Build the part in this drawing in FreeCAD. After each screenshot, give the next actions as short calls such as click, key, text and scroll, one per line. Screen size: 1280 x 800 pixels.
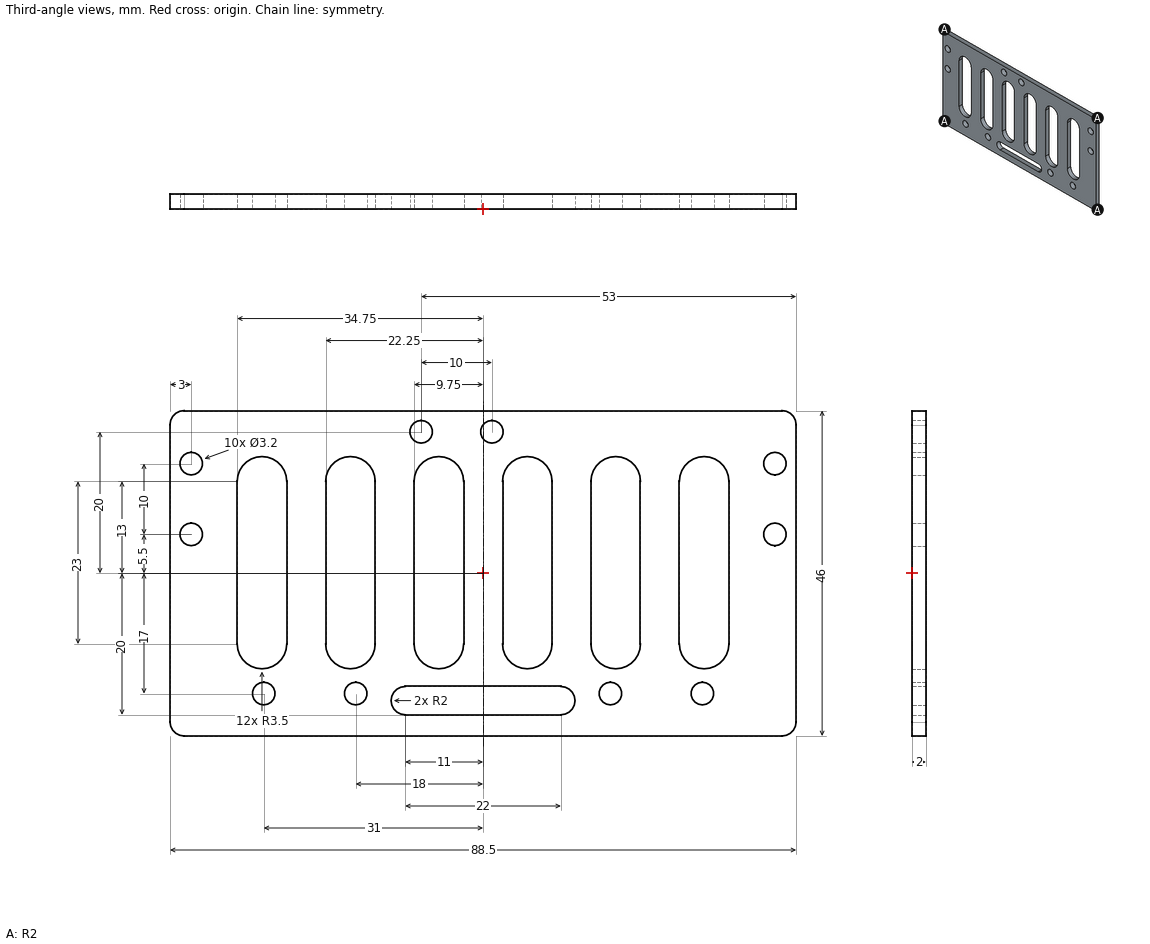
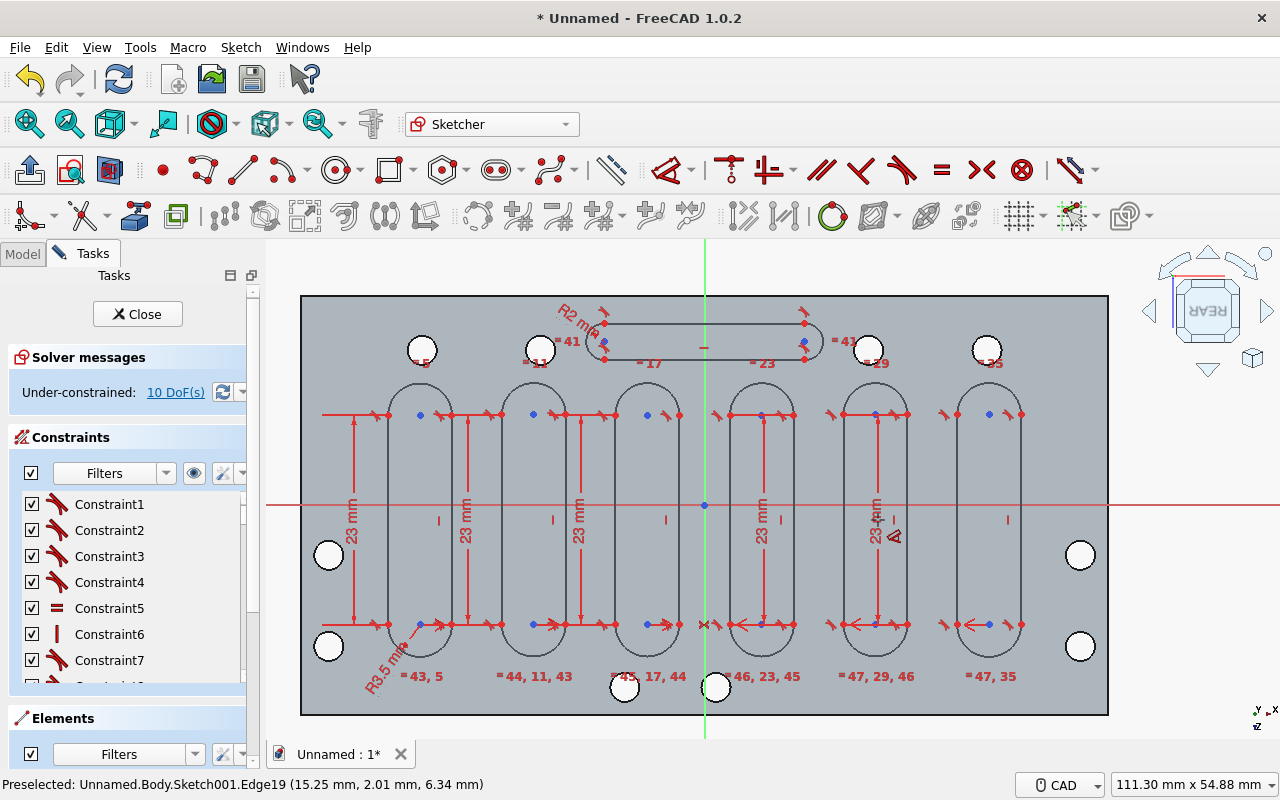
click(957, 562)
click(991, 520)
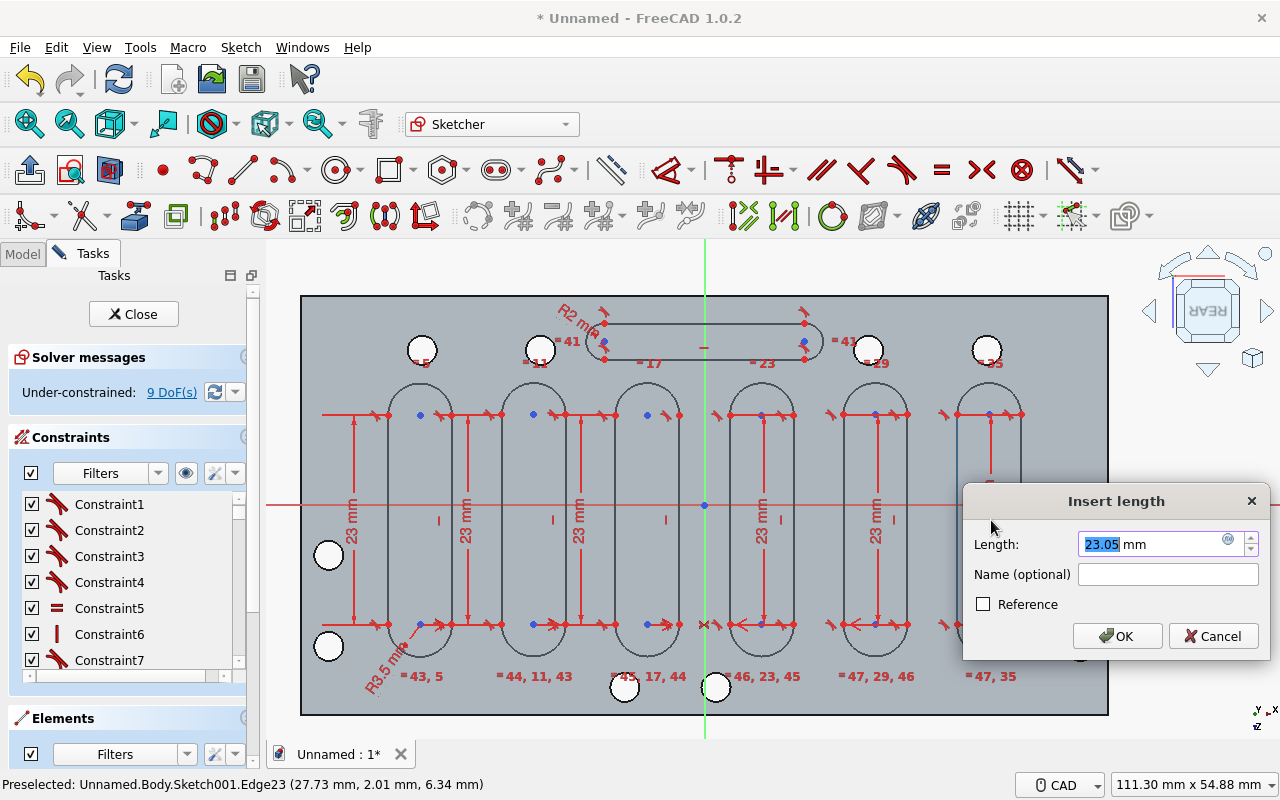
text(23)
key(Return)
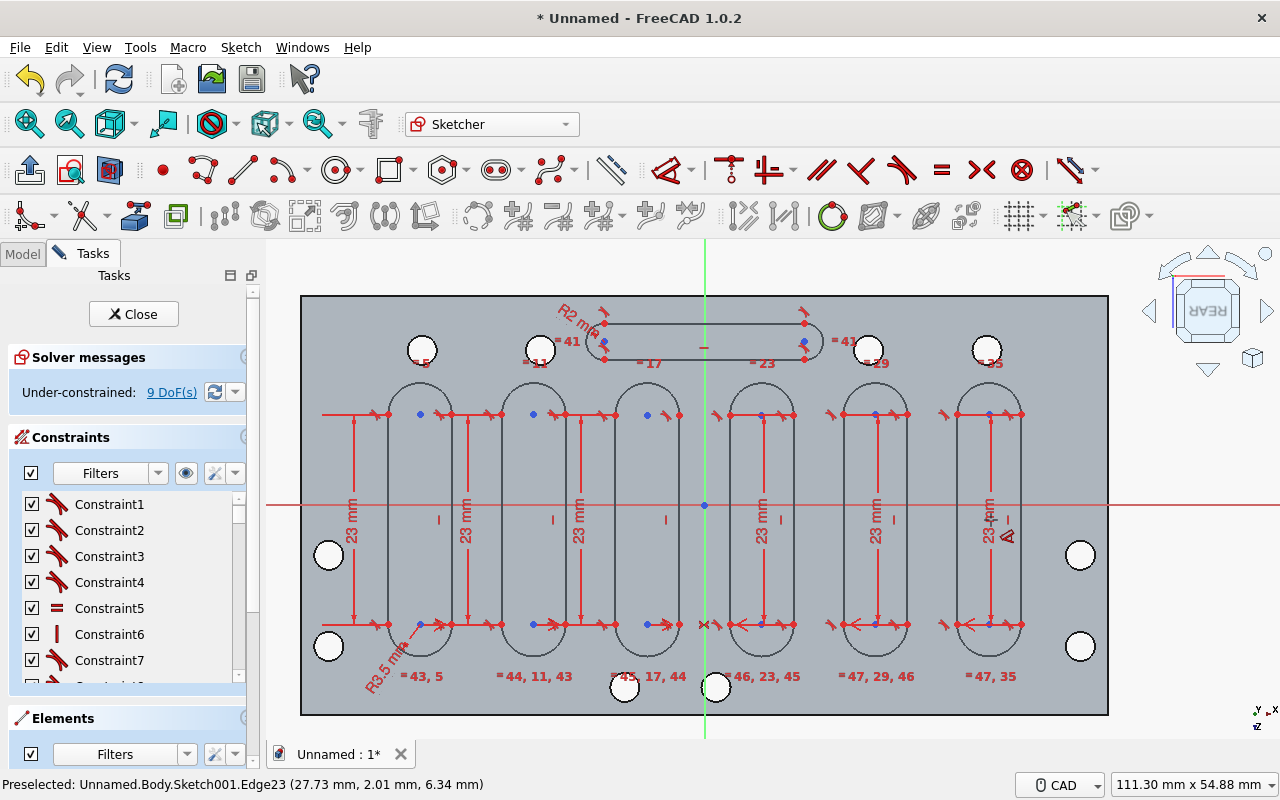
click(665, 324)
click(659, 290)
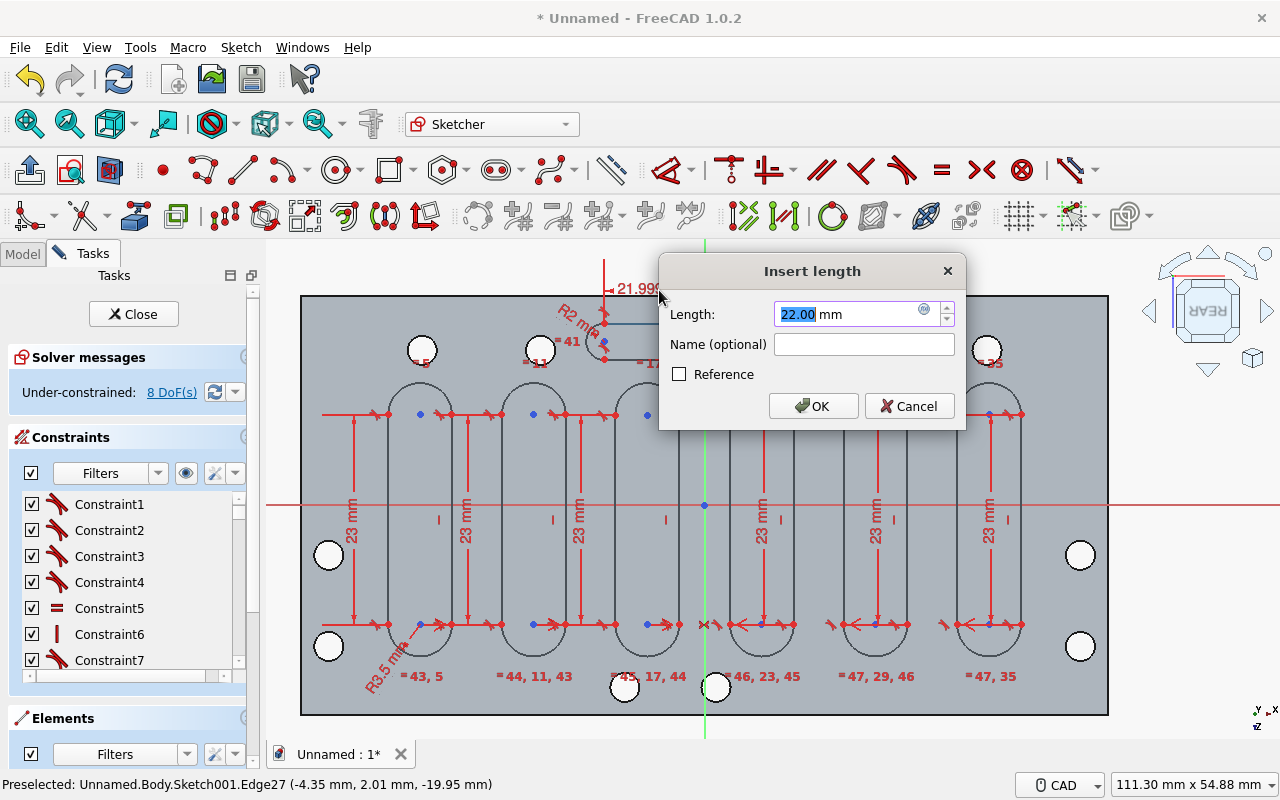
text(22)
key(Return)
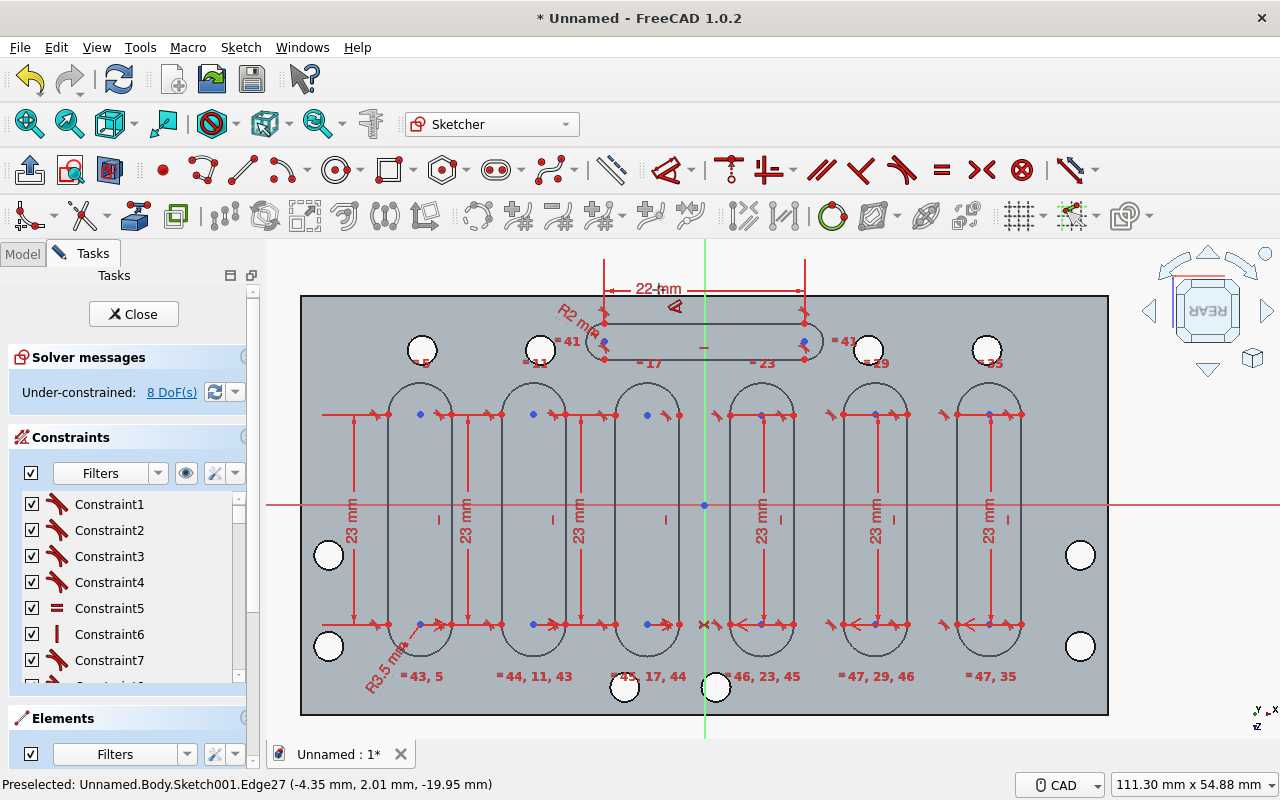
click(388, 625)
click(354, 565)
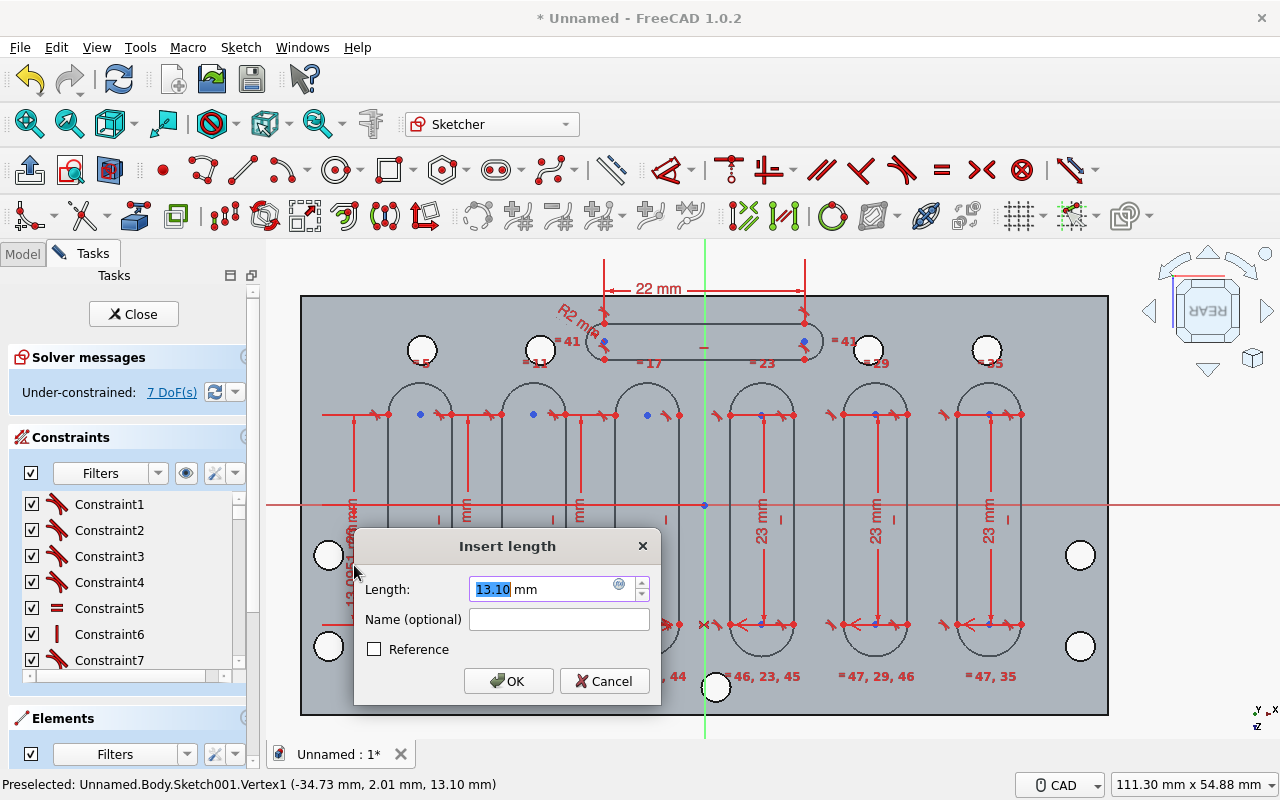
text(13)
key(Return)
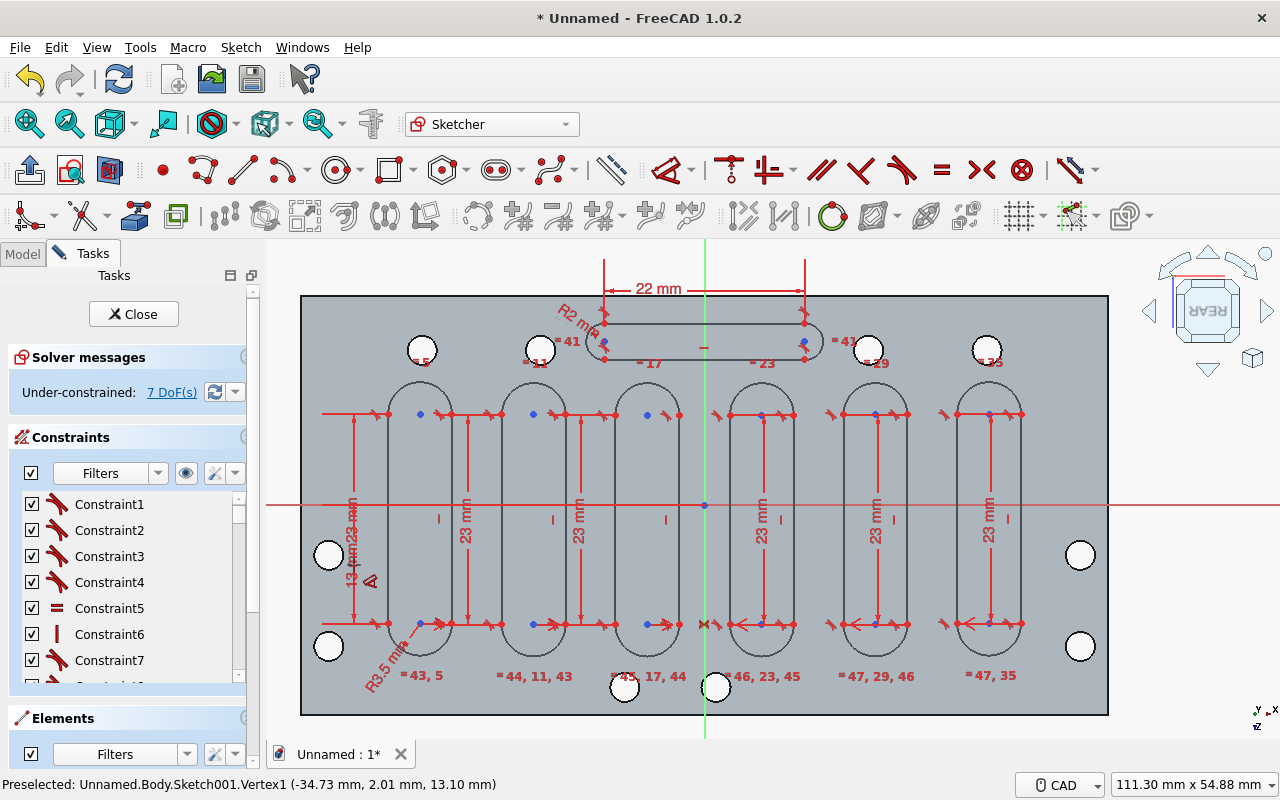
click(502, 625)
click(468, 565)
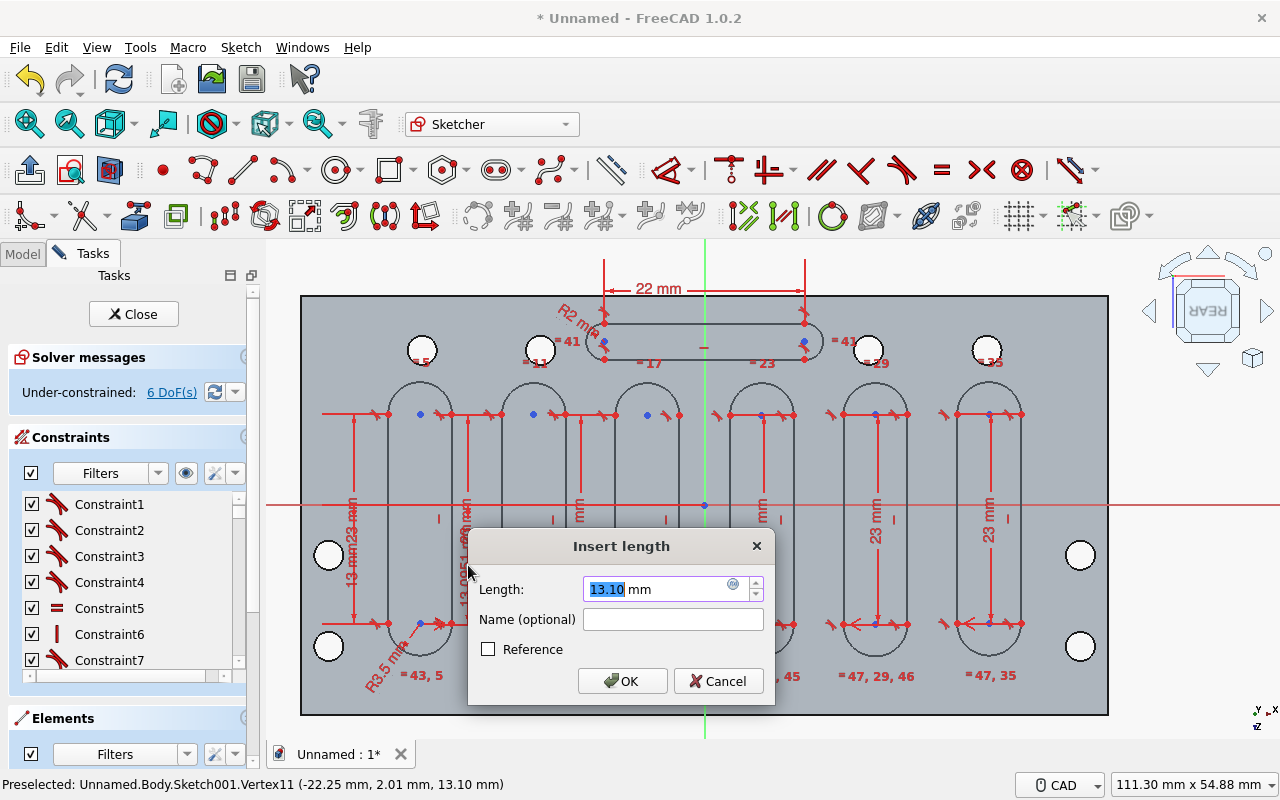
text(13)
key(Return)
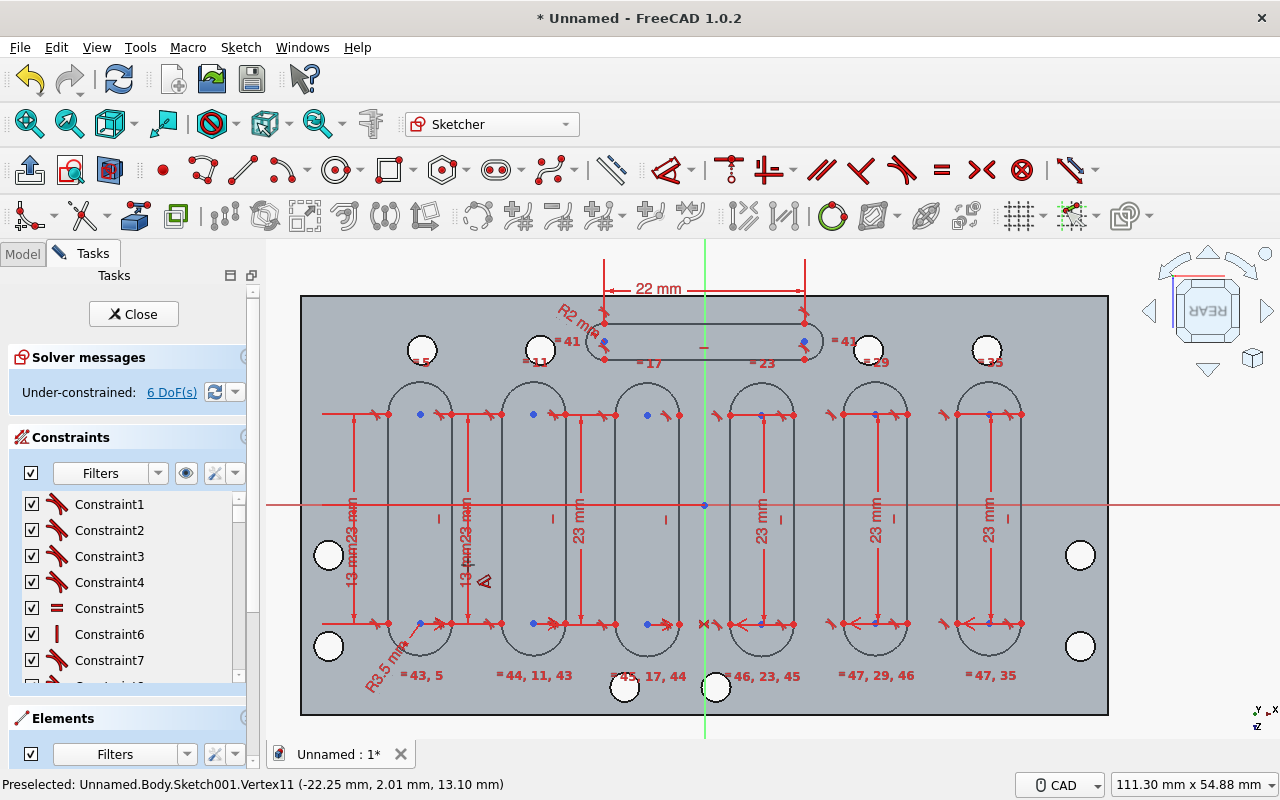
click(615, 625)
click(581, 565)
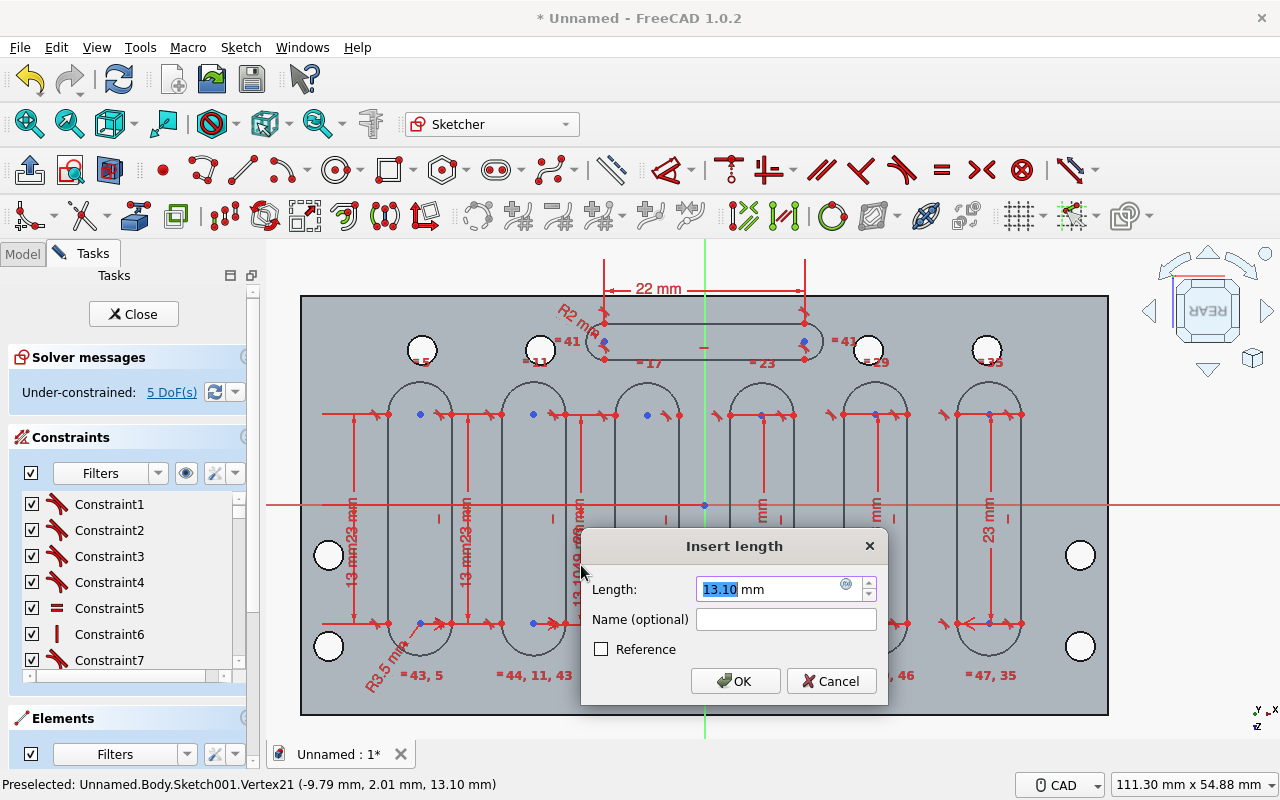
text(13)
key(Return)